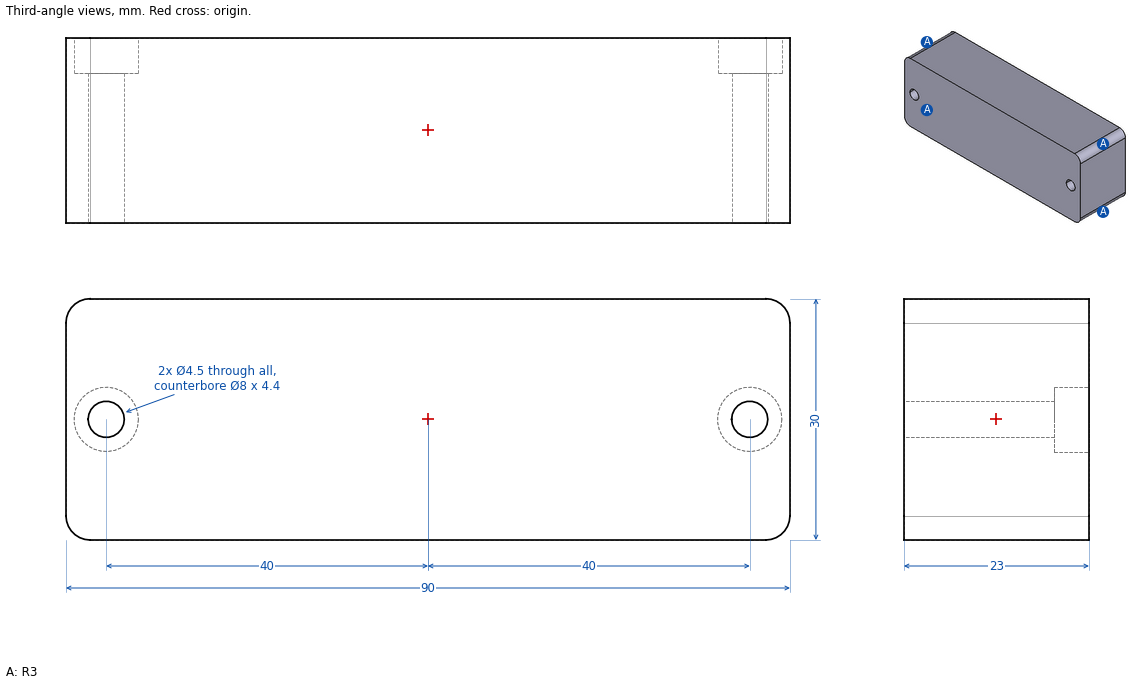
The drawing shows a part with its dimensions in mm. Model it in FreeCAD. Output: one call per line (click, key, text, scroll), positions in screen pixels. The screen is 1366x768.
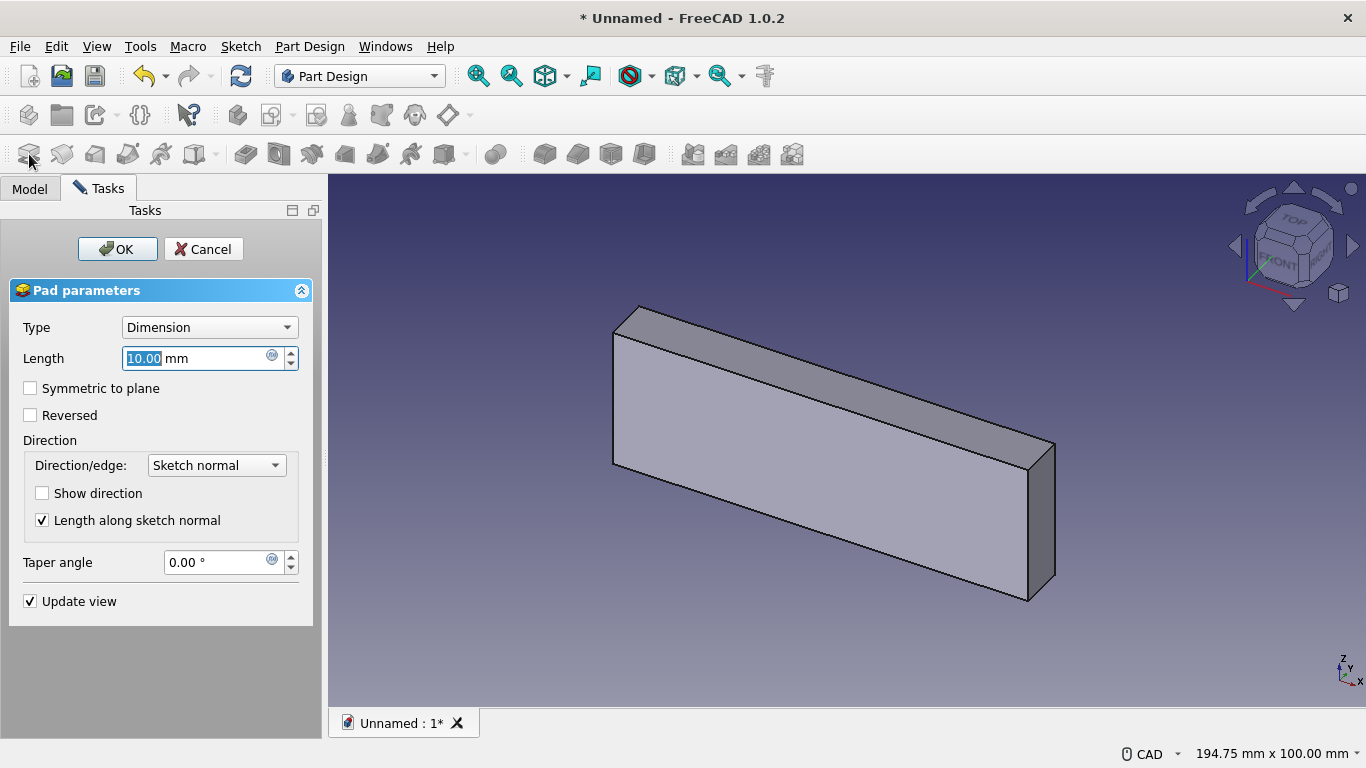
text(23)
key(Tab)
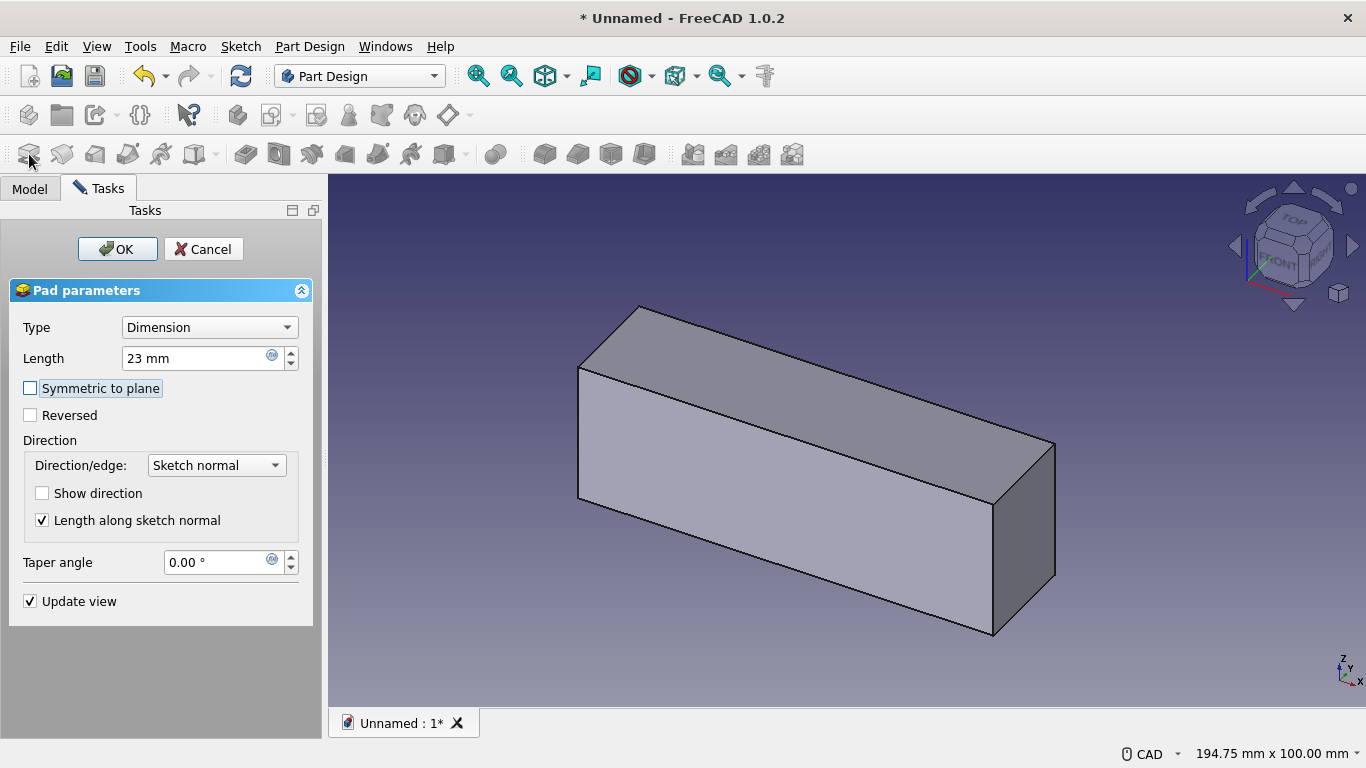
click(31, 388)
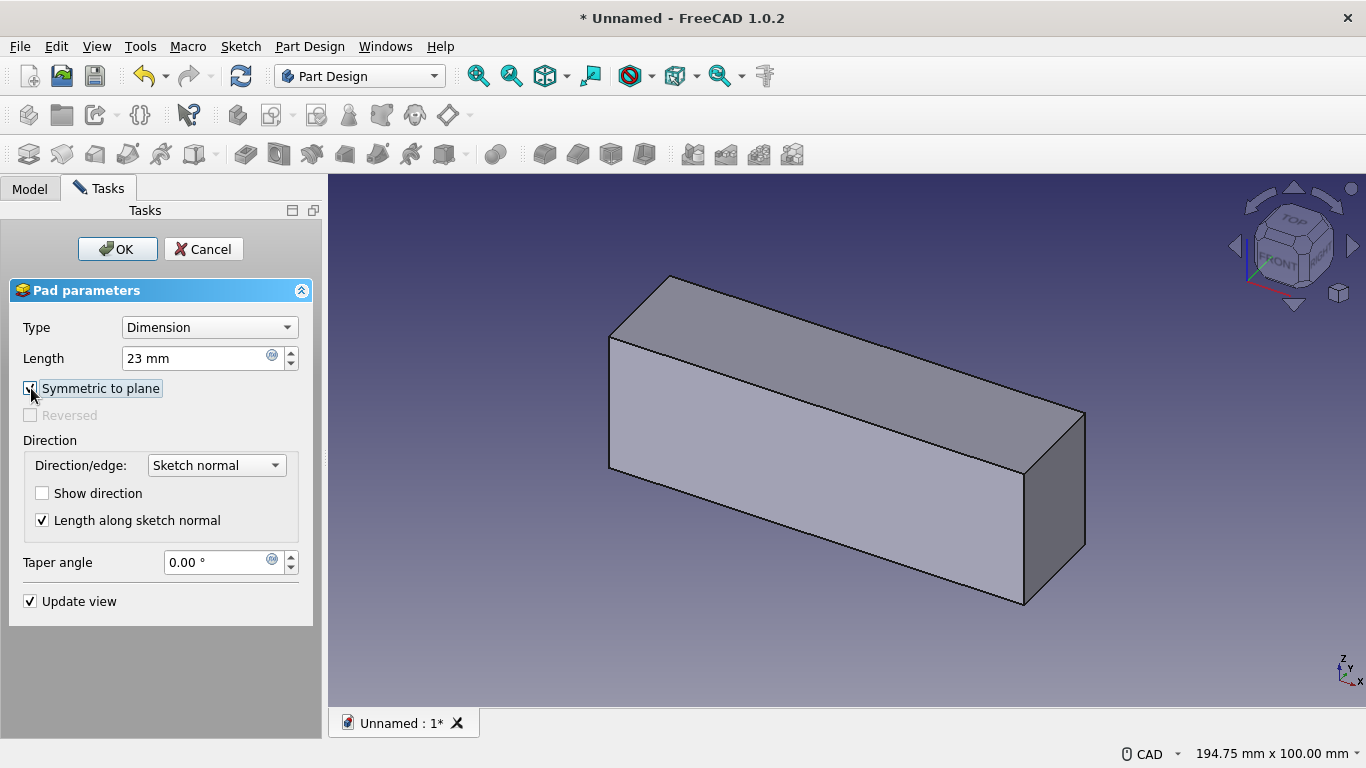
click(118, 249)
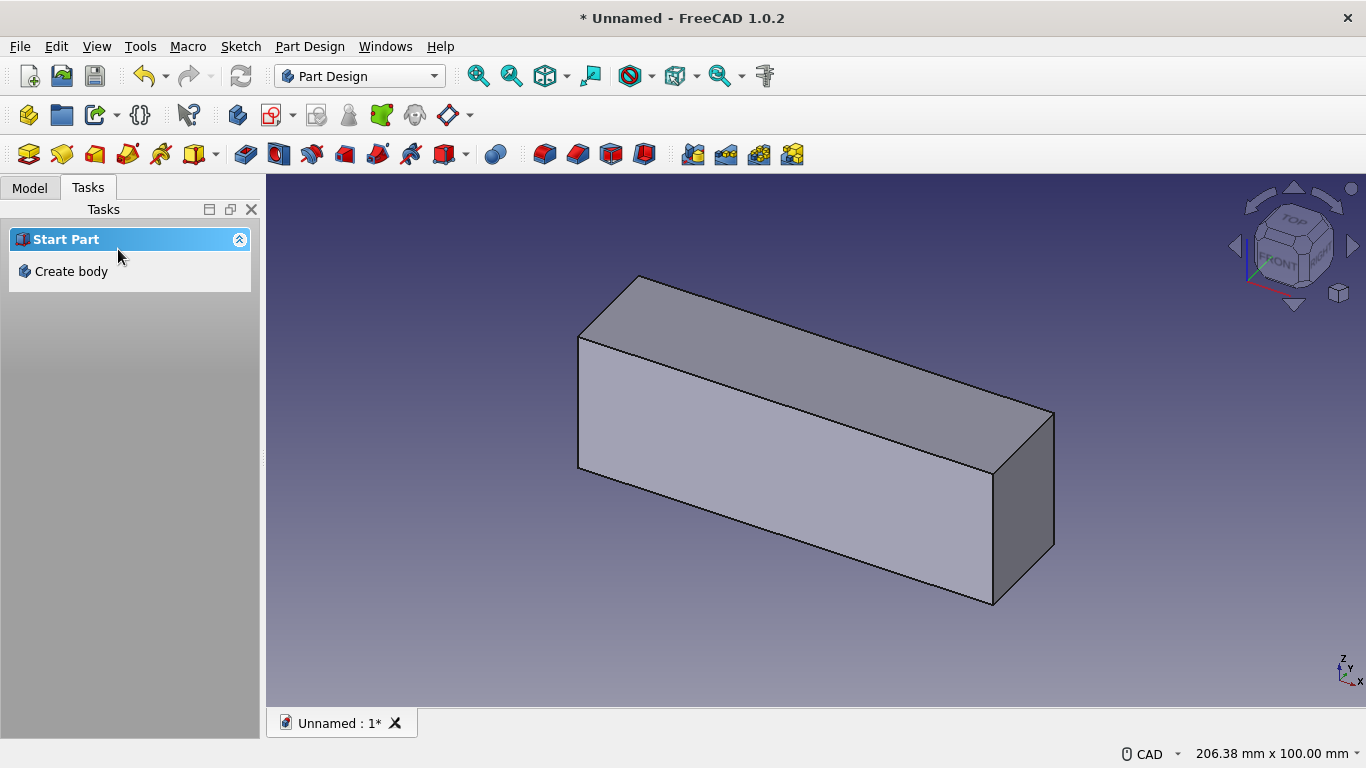
key(4)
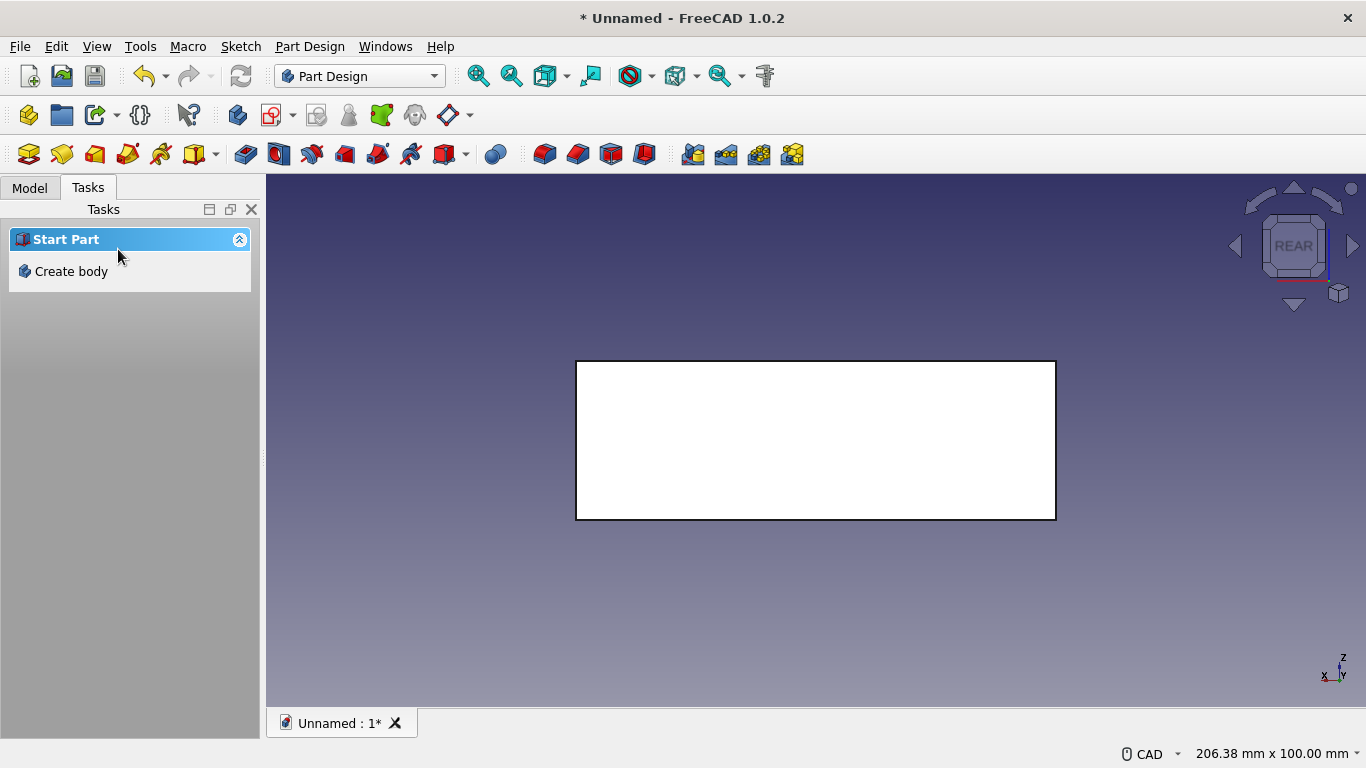
key(v)
key(f)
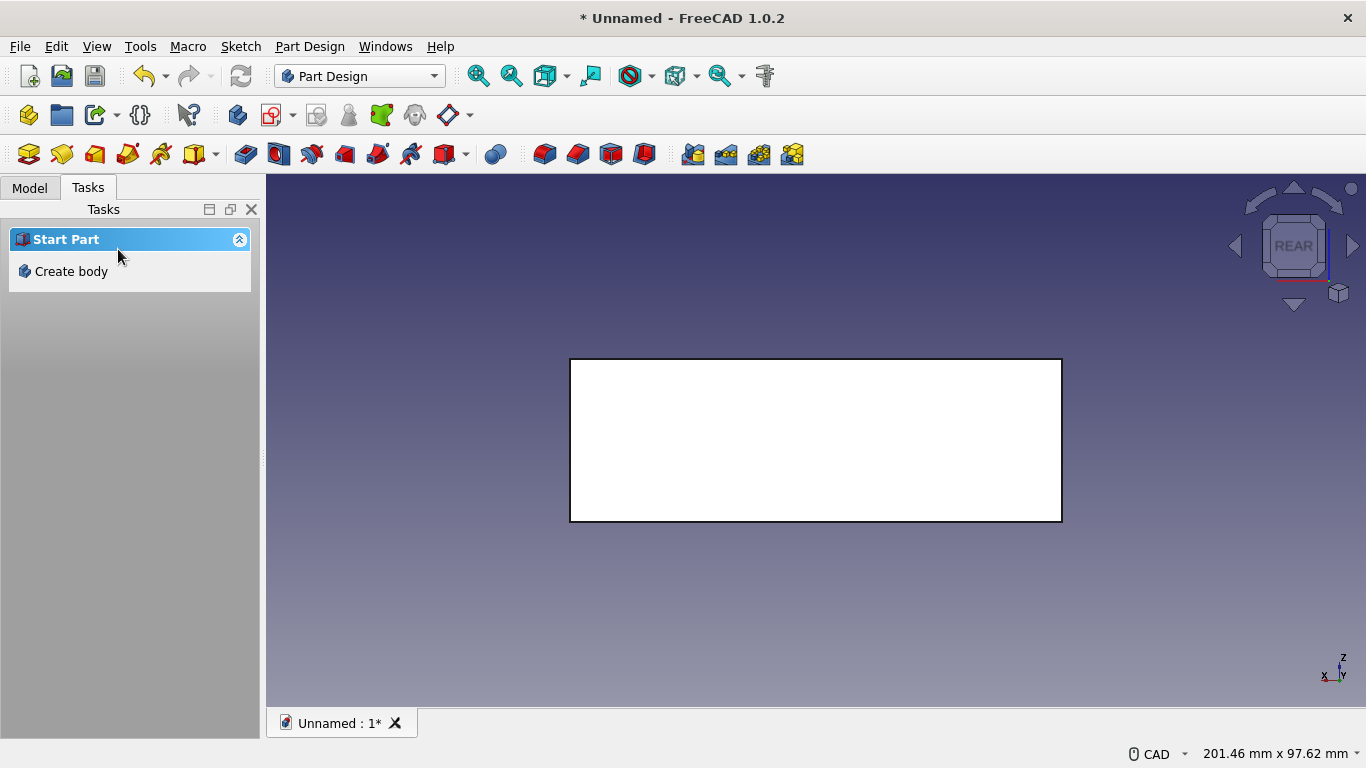
click(676, 440)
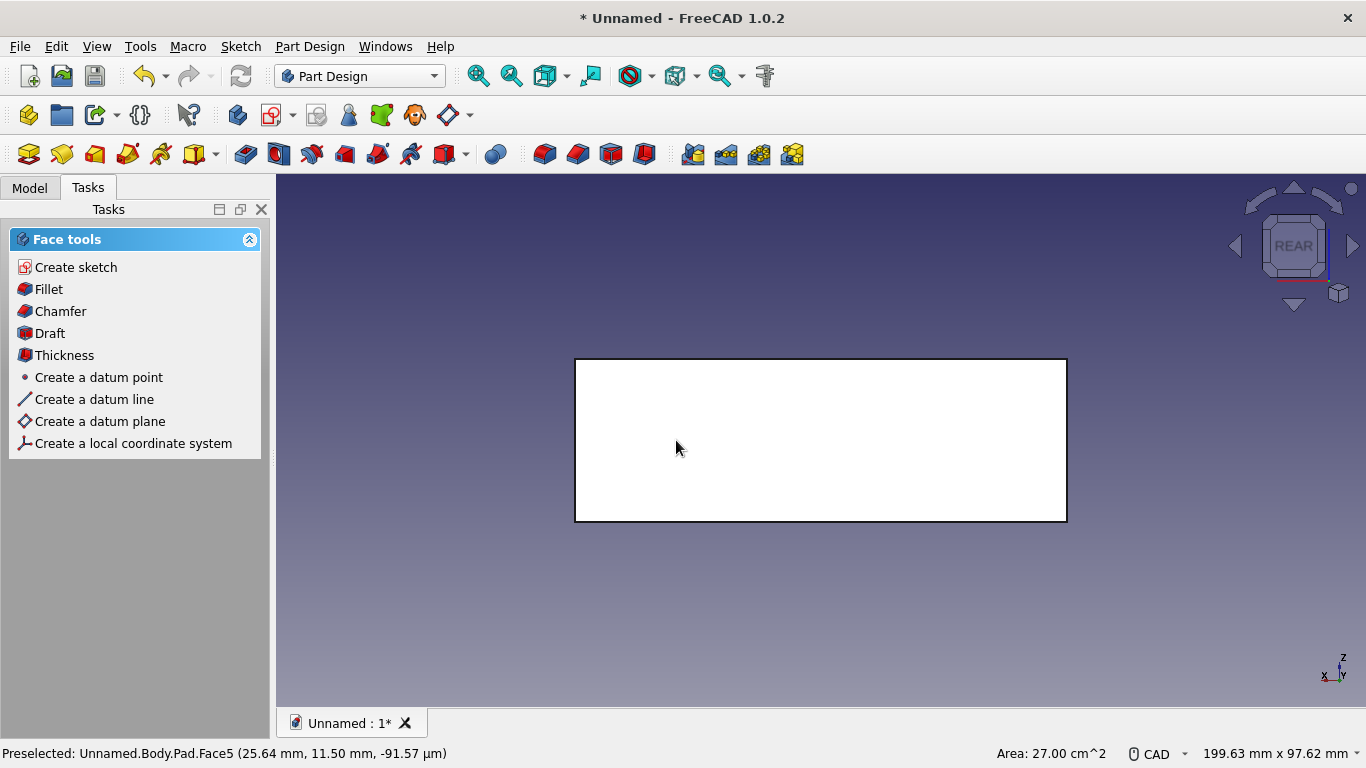
click(270, 116)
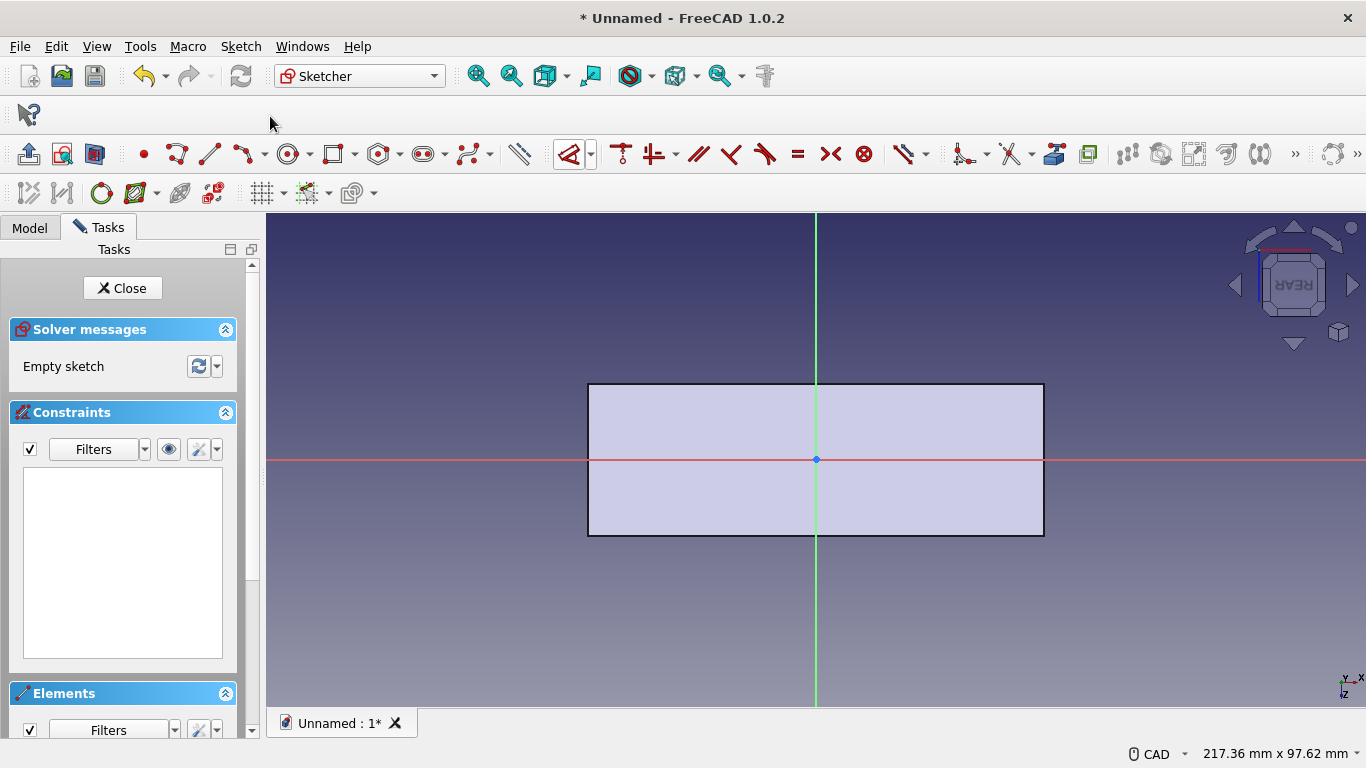
scroll(955, 460, up, 2)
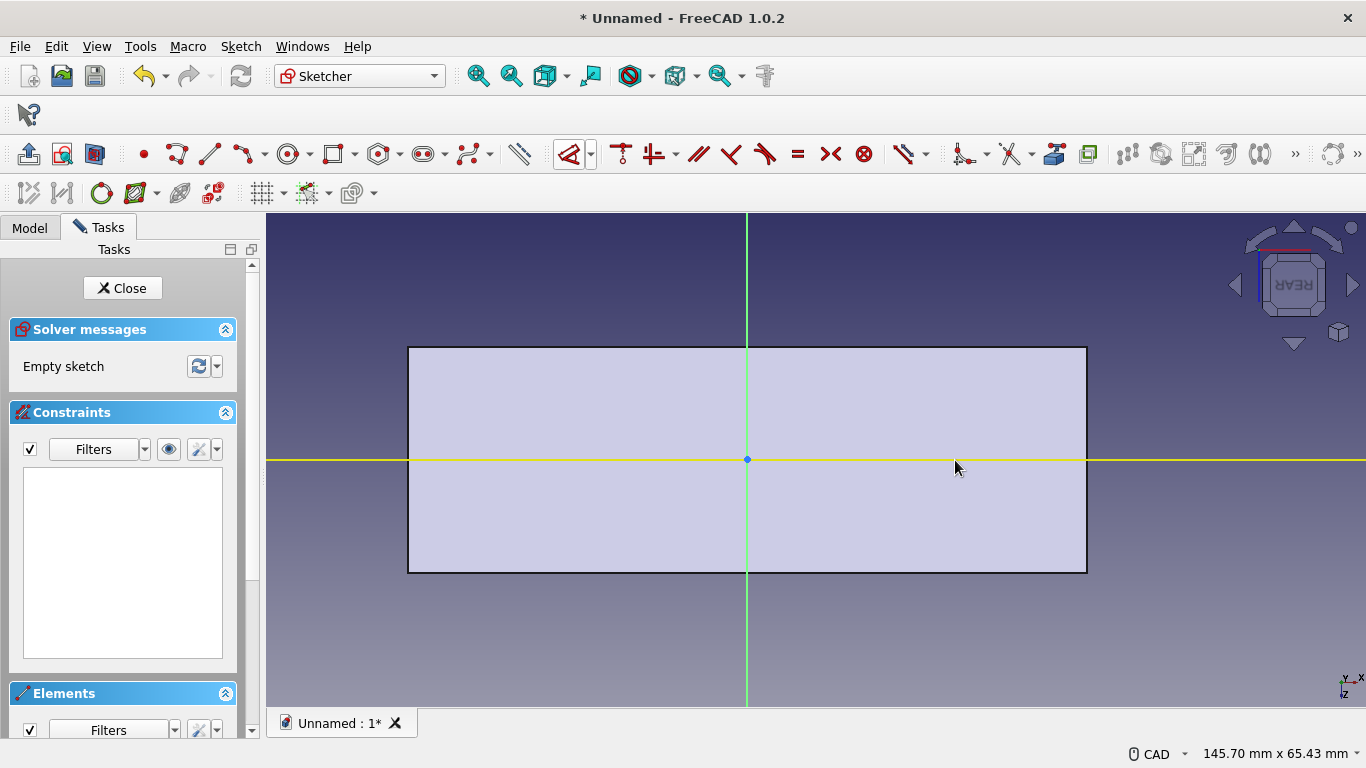
key(g)
key(c)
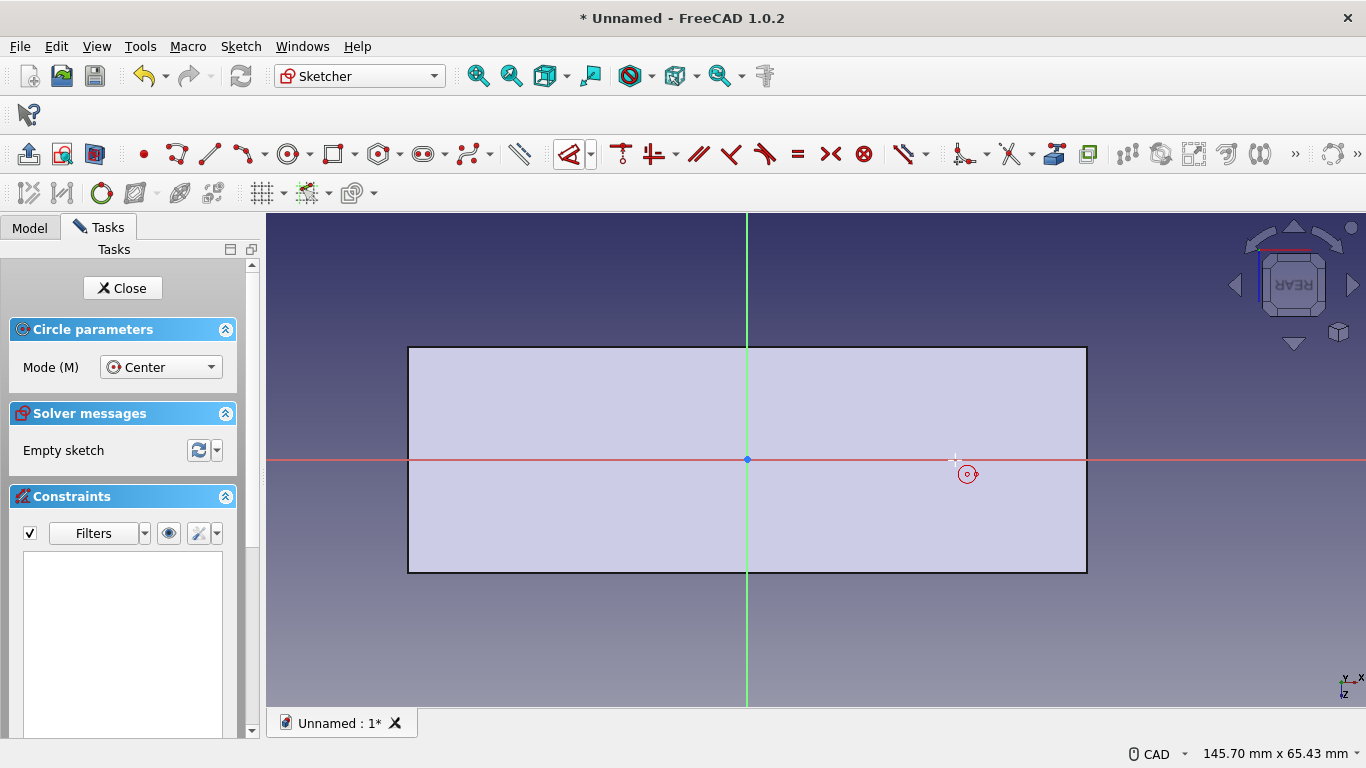
scroll(445, 460, up, 2)